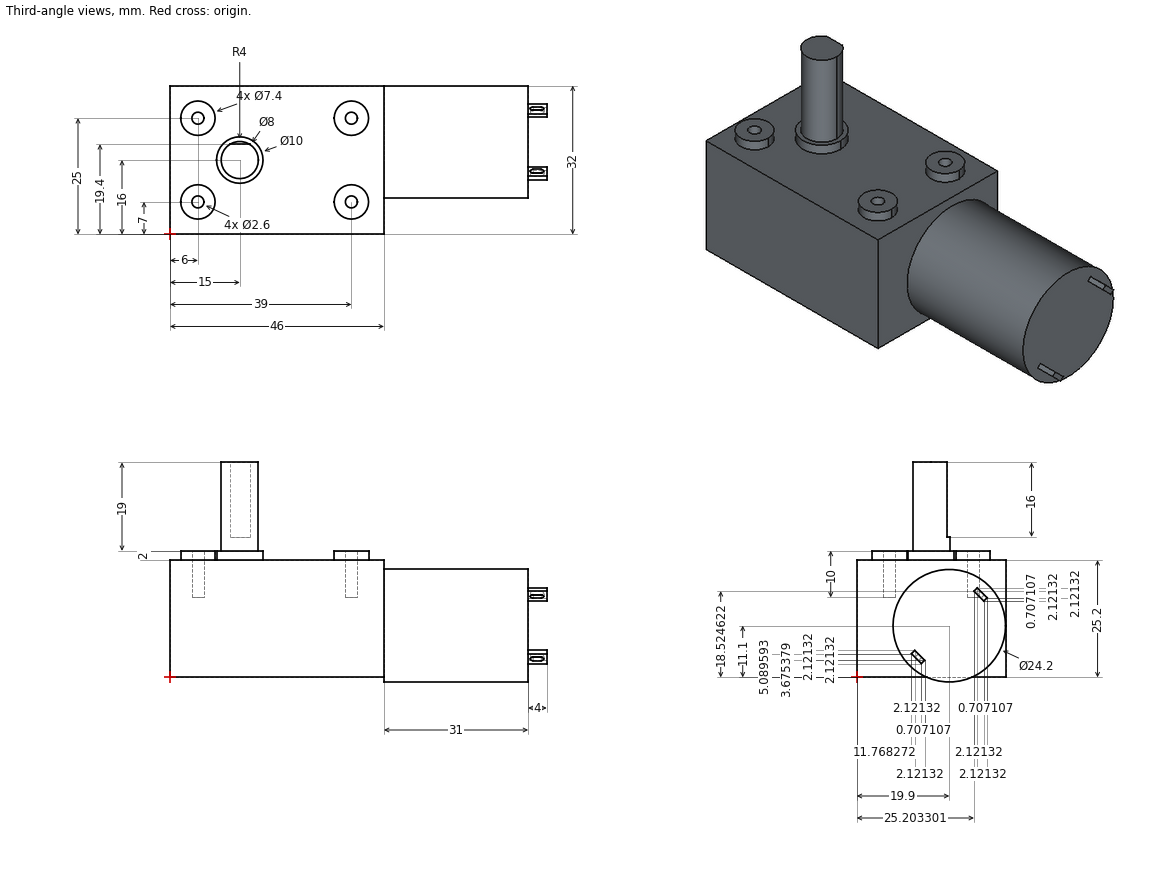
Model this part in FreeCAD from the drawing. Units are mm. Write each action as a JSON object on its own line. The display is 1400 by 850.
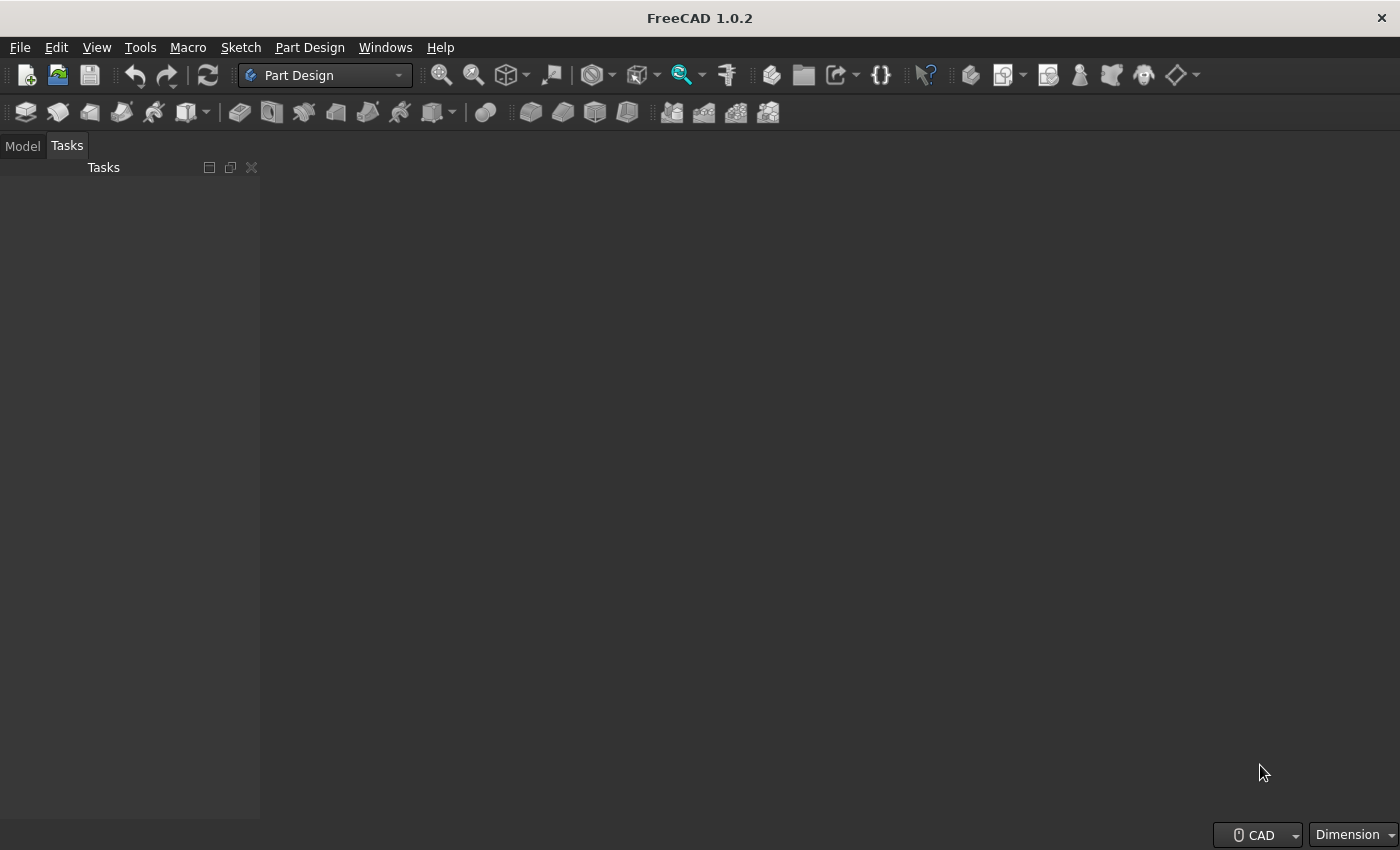
{"action": "left_click", "coordinate": [26, 76]}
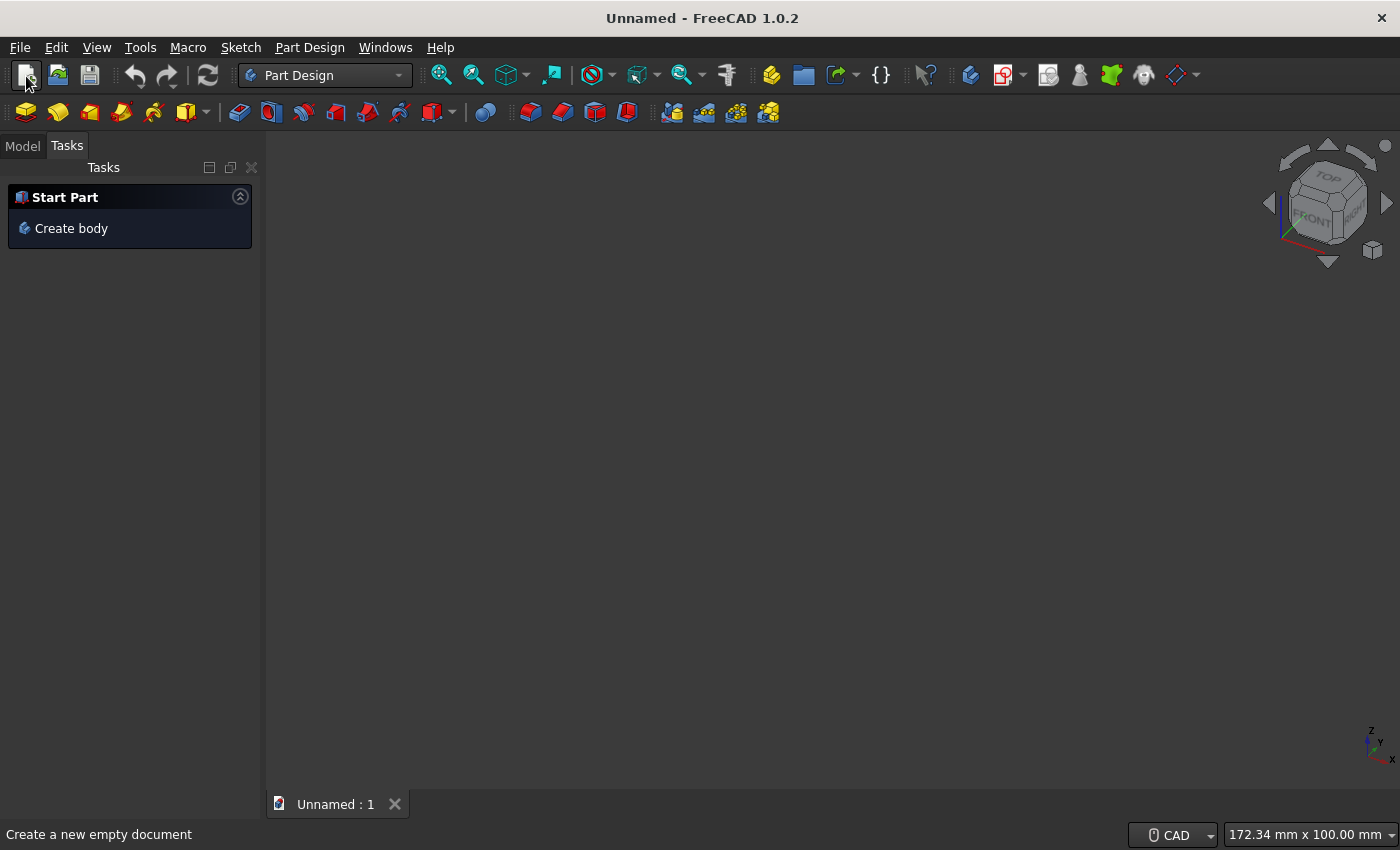
{"action": "left_click", "coordinate": [1004, 76]}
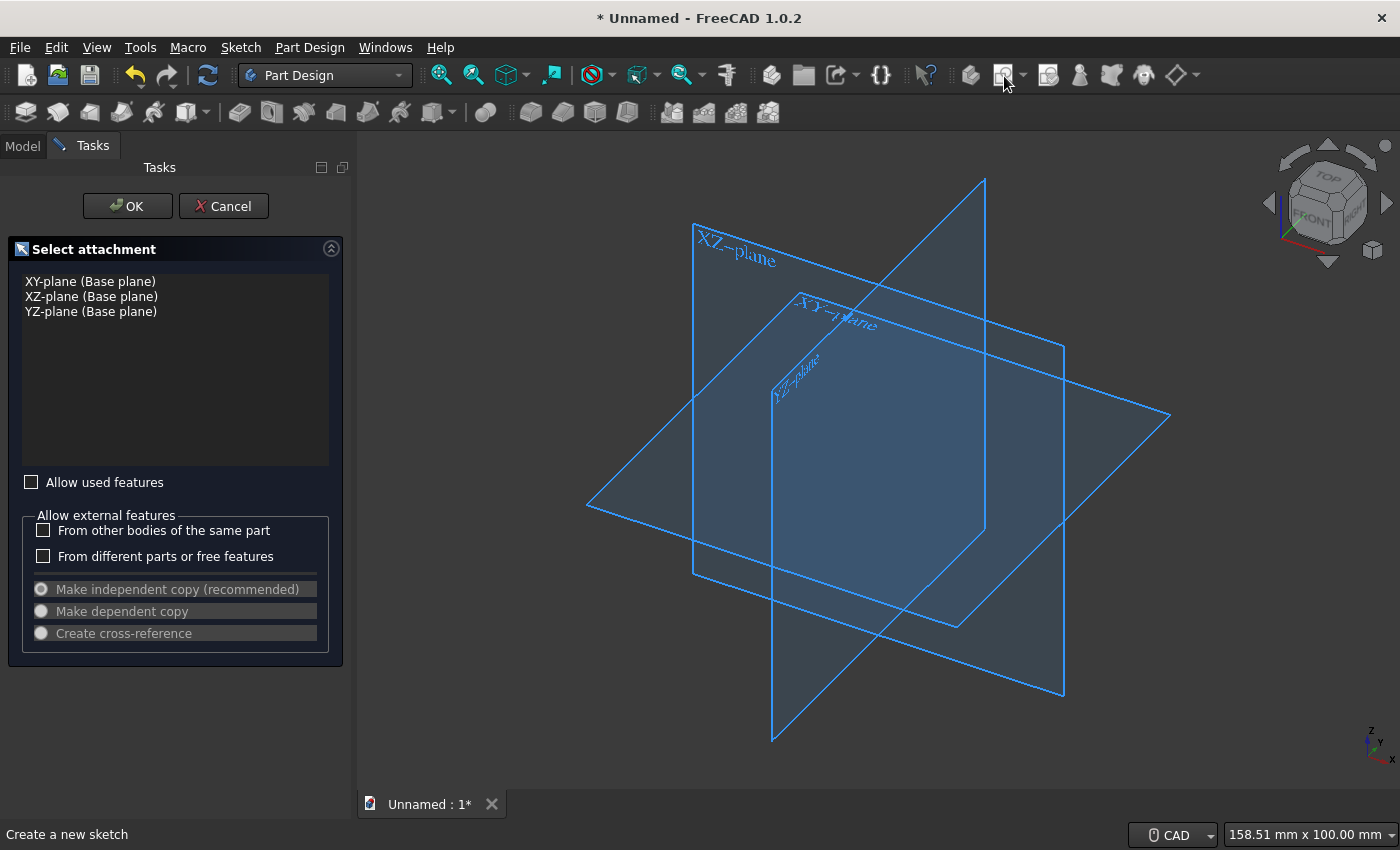
{"action": "left_click", "coordinate": [82, 282]}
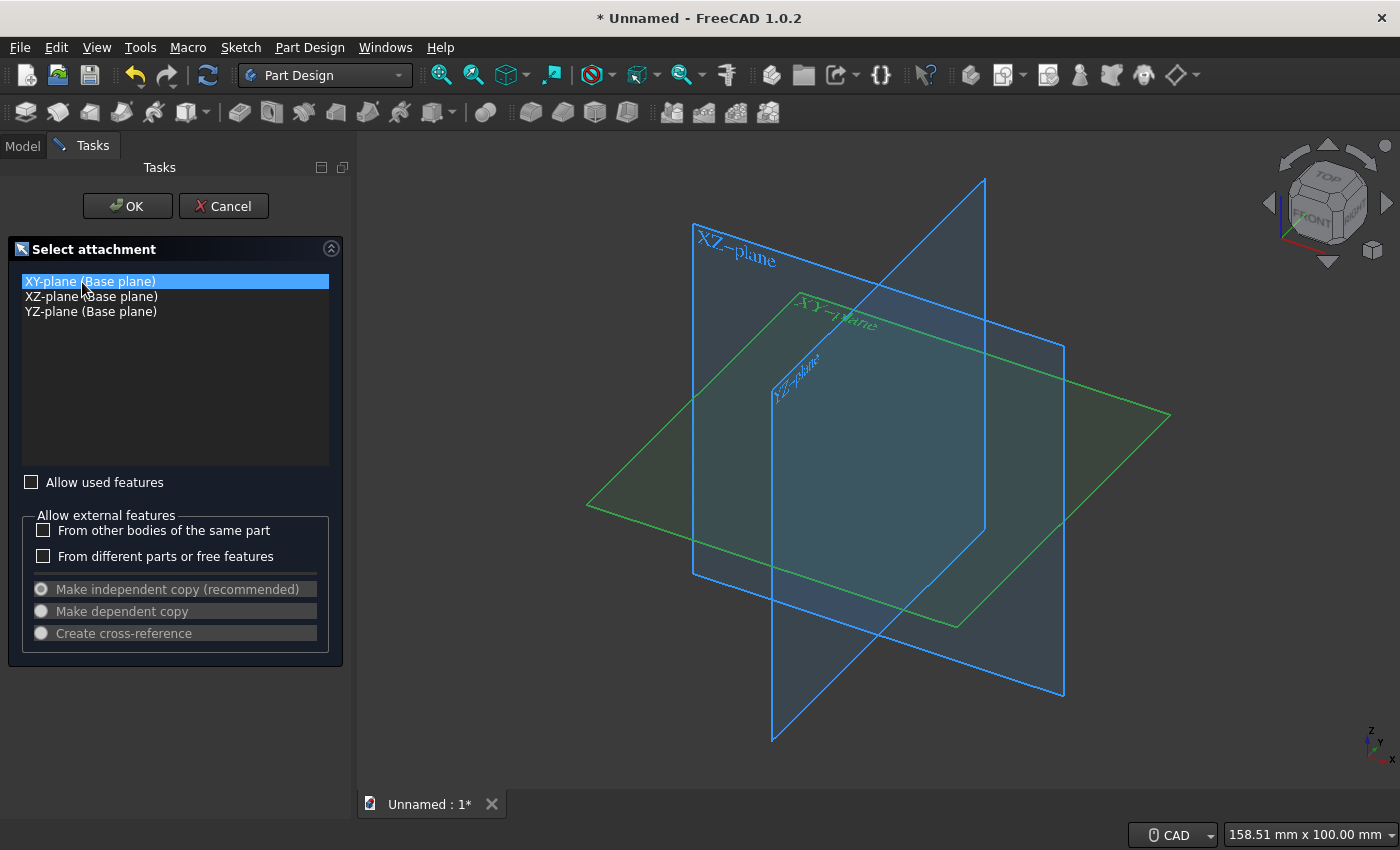
{"action": "left_click", "coordinate": [128, 206]}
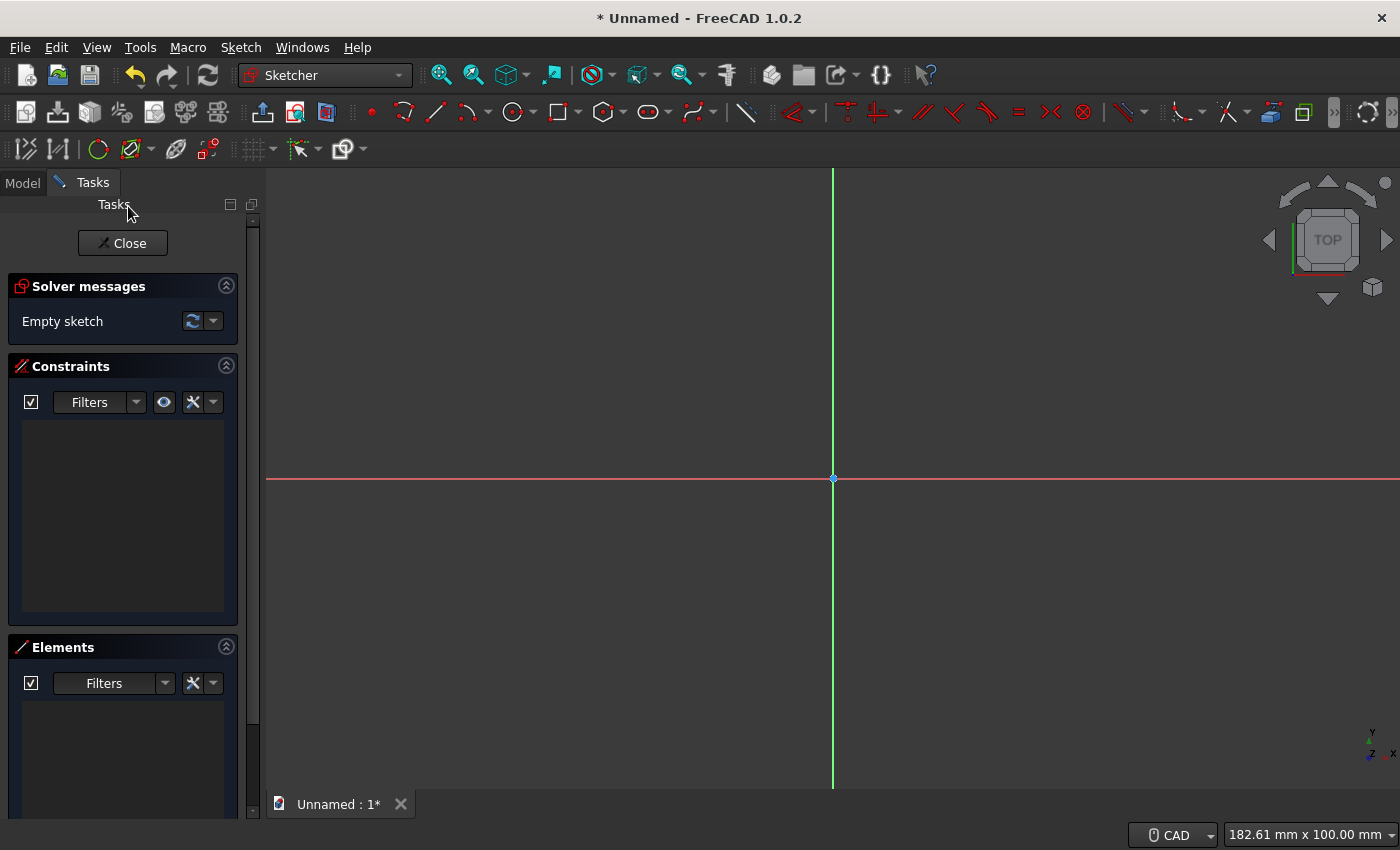
{"action": "scroll", "coordinate": [1233, 258], "scroll_direction": "up", "scroll_amount": 3}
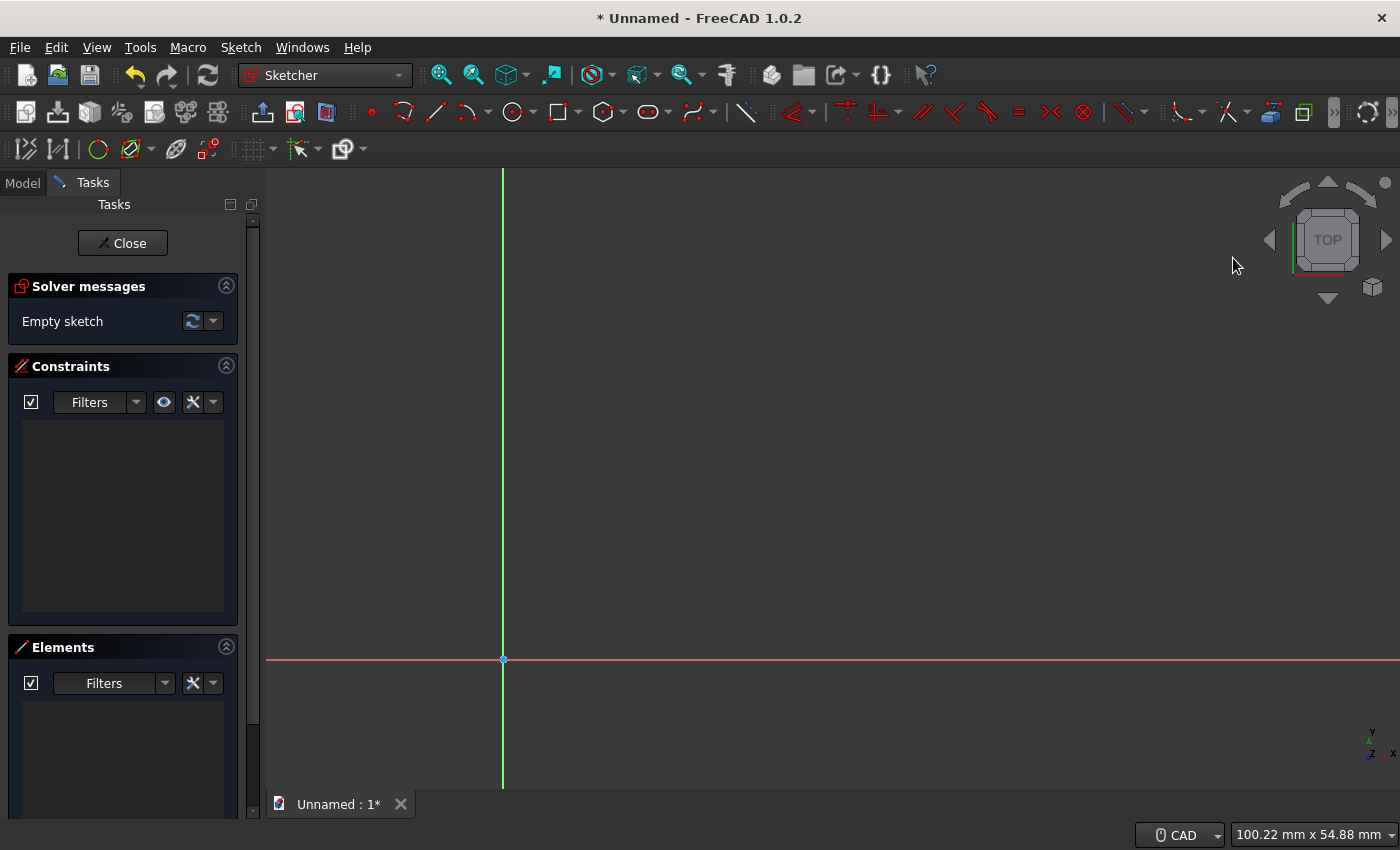
{"action": "left_click", "coordinate": [558, 112]}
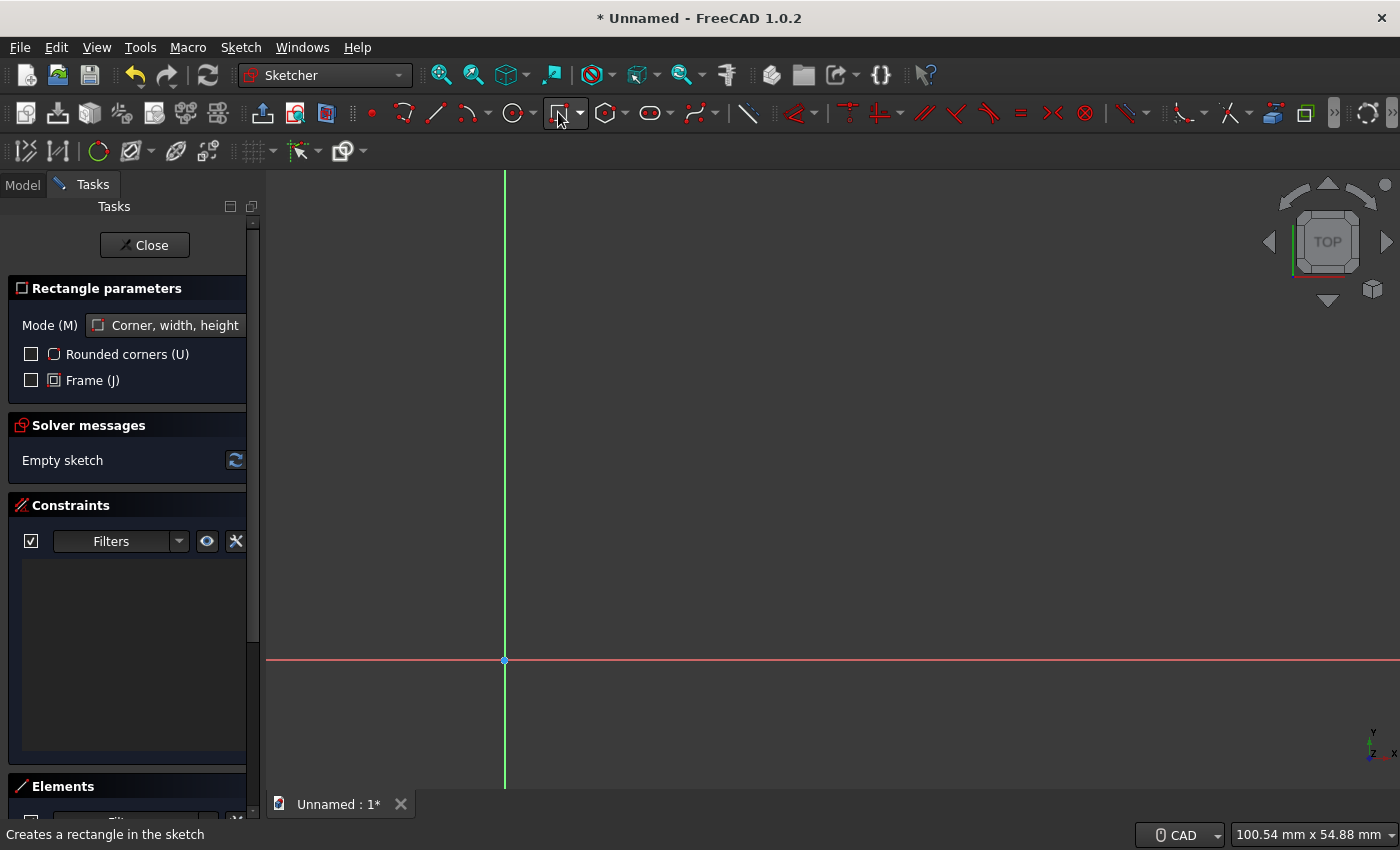
{"action": "left_click", "coordinate": [505, 660]}
{"action": "mouse_move", "coordinate": [1023, 299]}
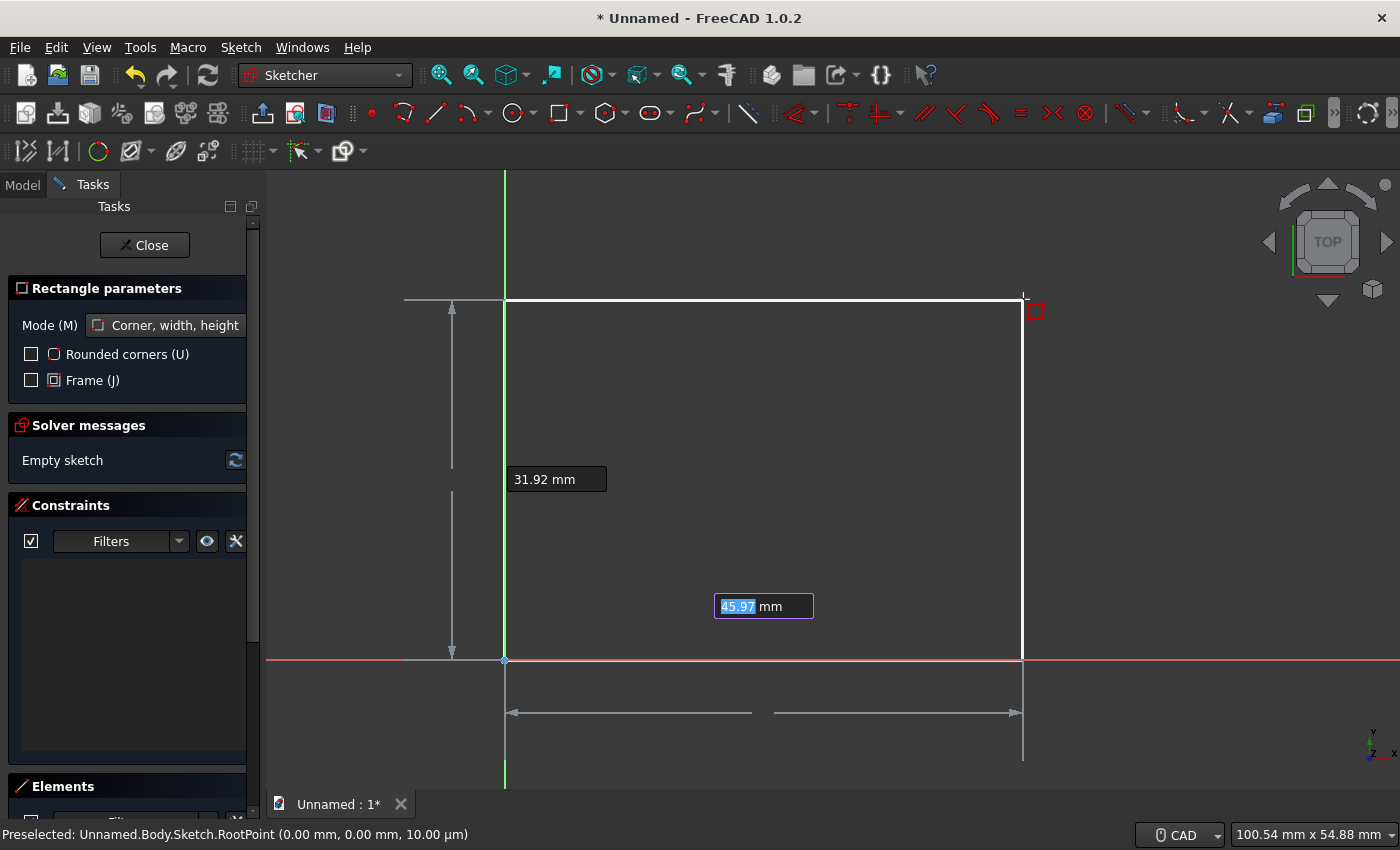
{"action": "type", "text": "46"}
{"action": "key", "text": "Tab"}
{"action": "type", "text": "32"}
{"action": "key", "text": "Return"}
{"action": "key", "text": "Escape"}